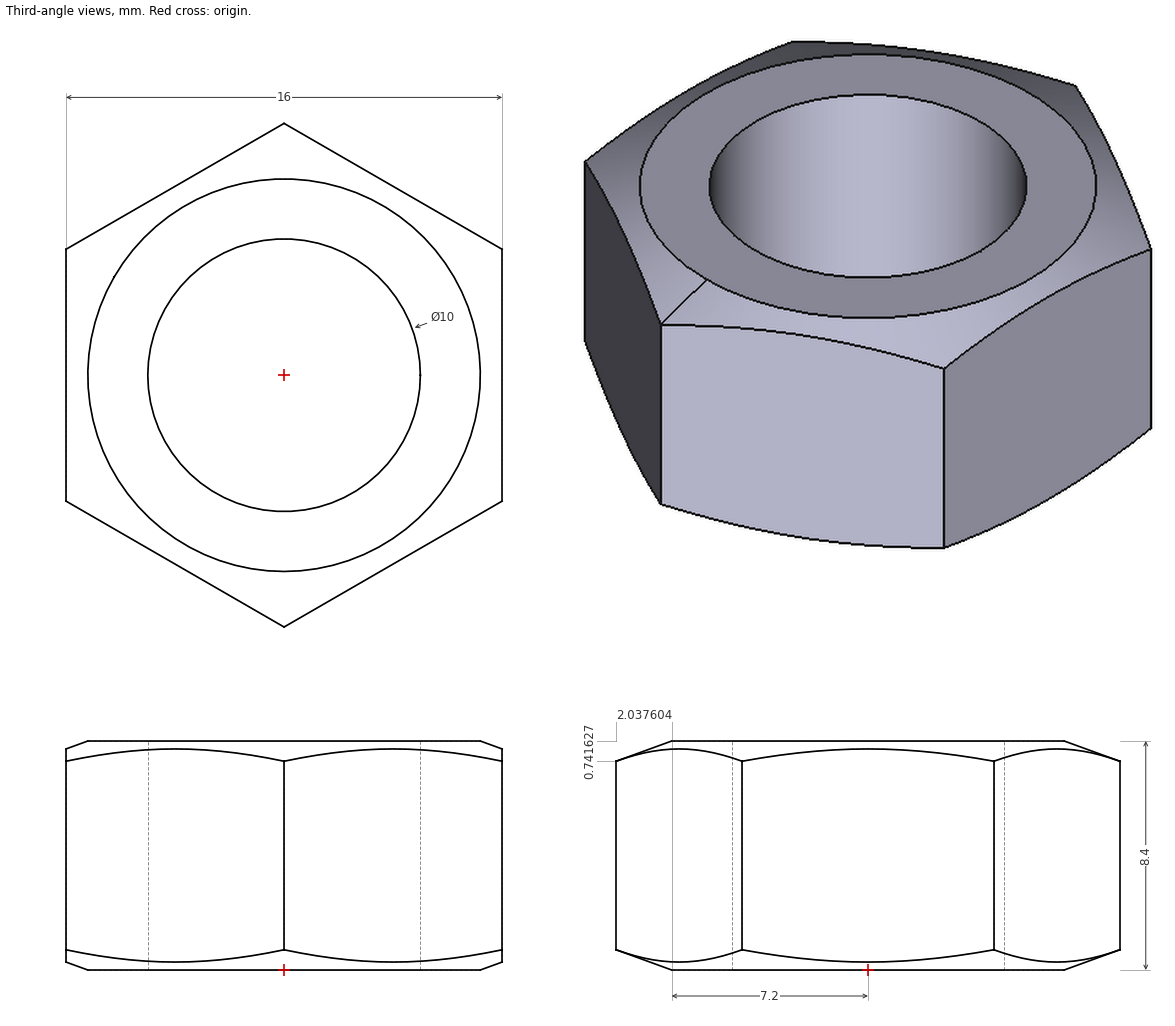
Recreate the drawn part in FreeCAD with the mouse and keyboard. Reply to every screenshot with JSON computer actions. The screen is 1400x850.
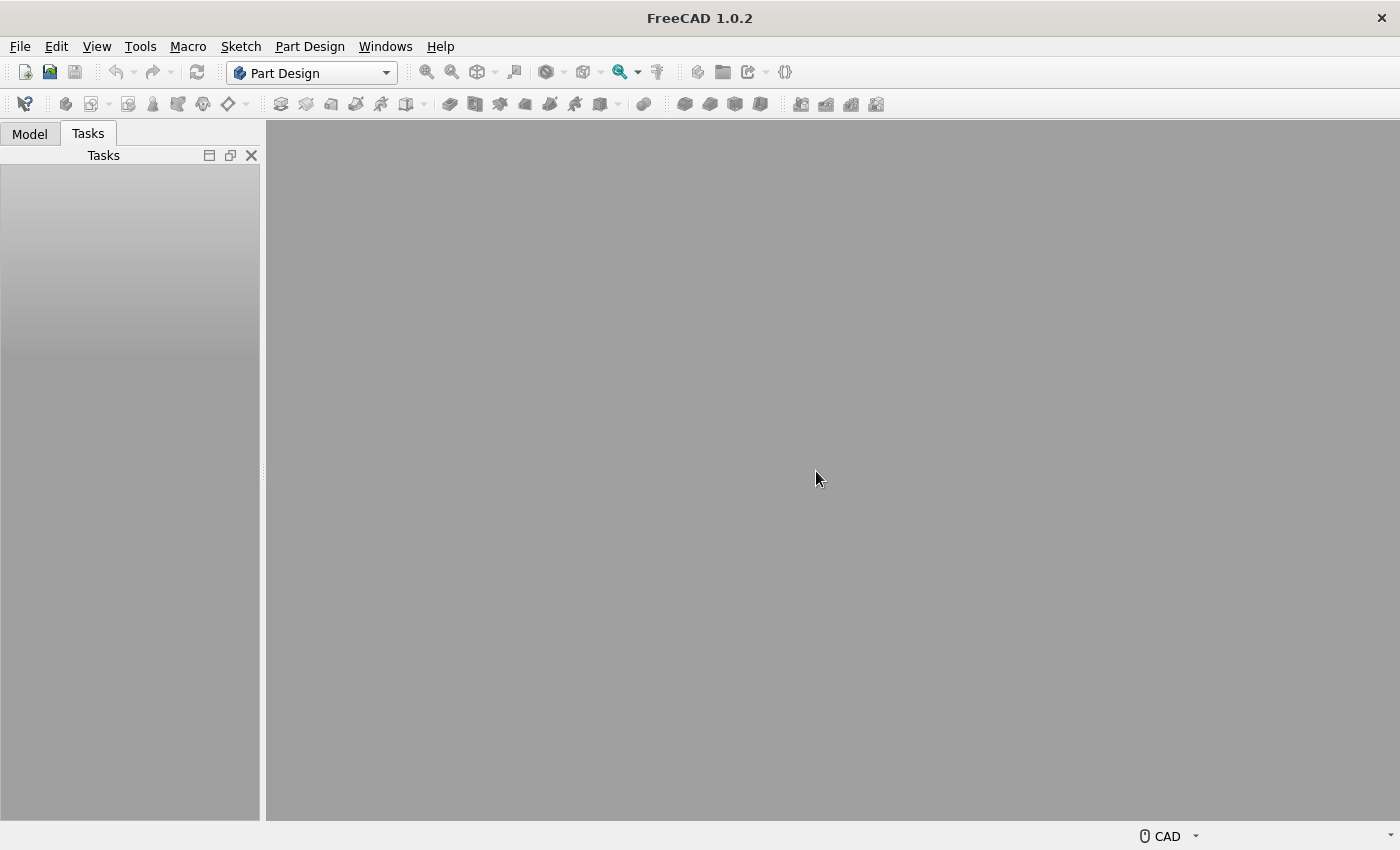
{"action": "left_click", "coordinate": [25, 72]}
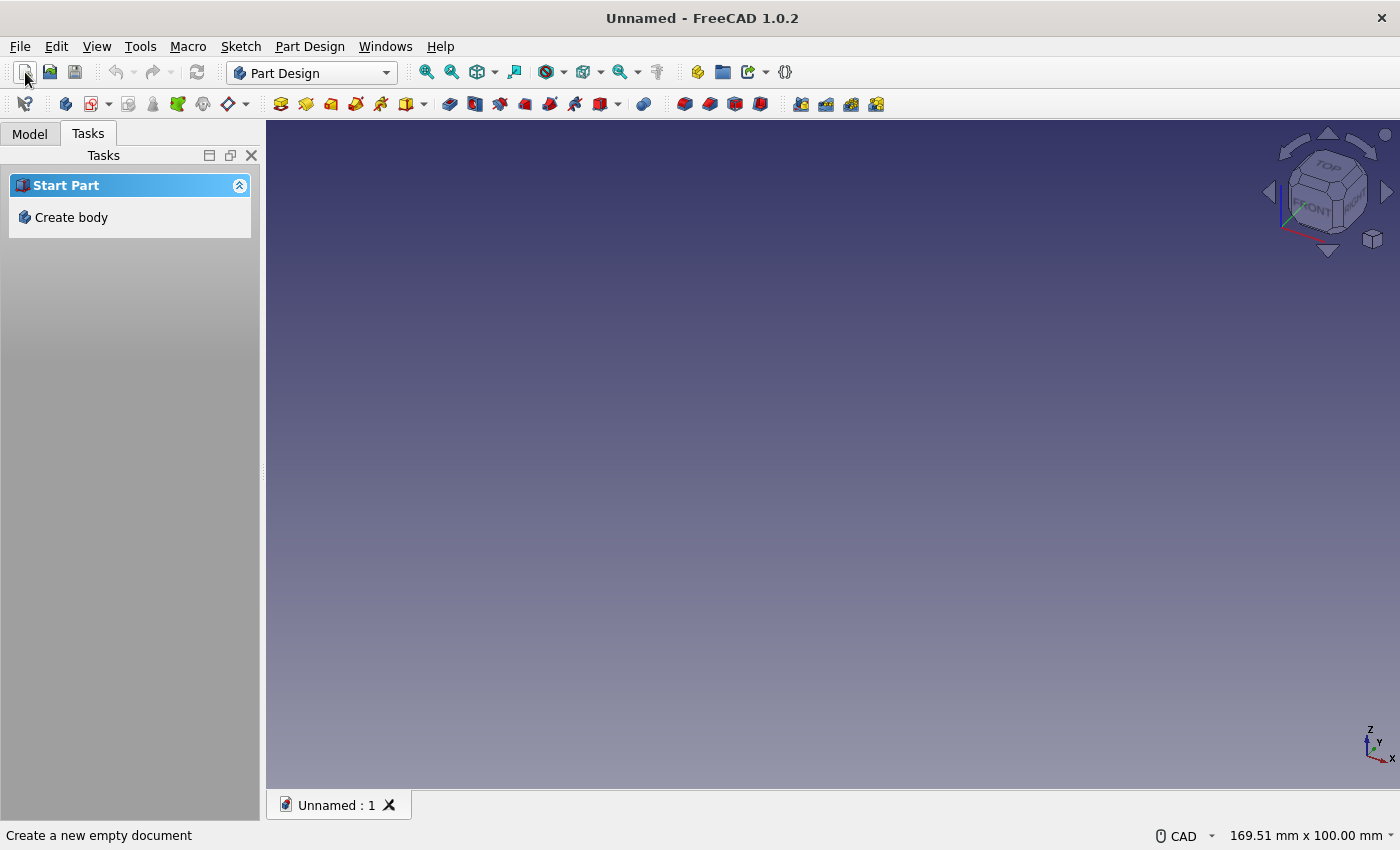
{"action": "left_click", "coordinate": [90, 104]}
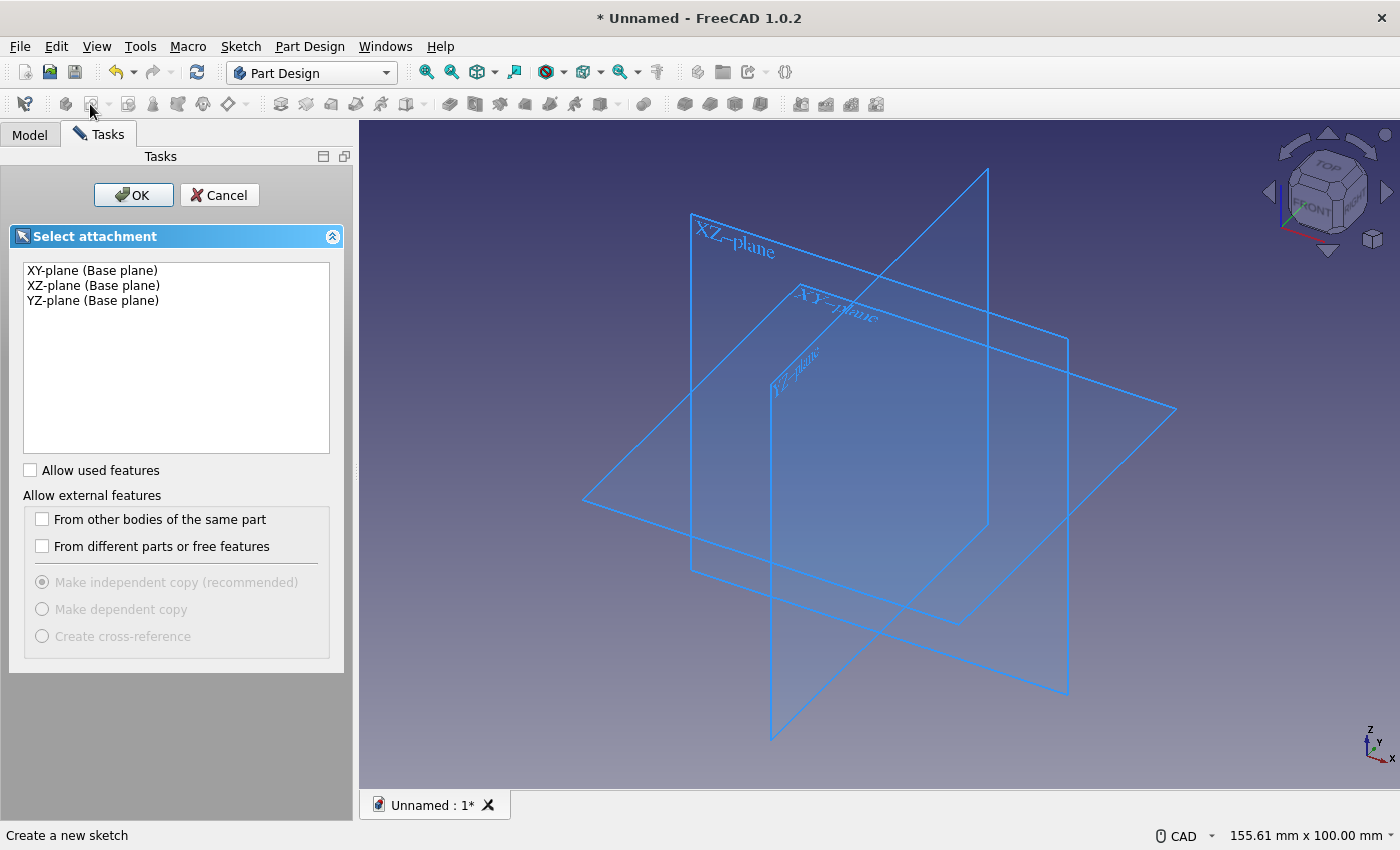
{"action": "left_click", "coordinate": [84, 270]}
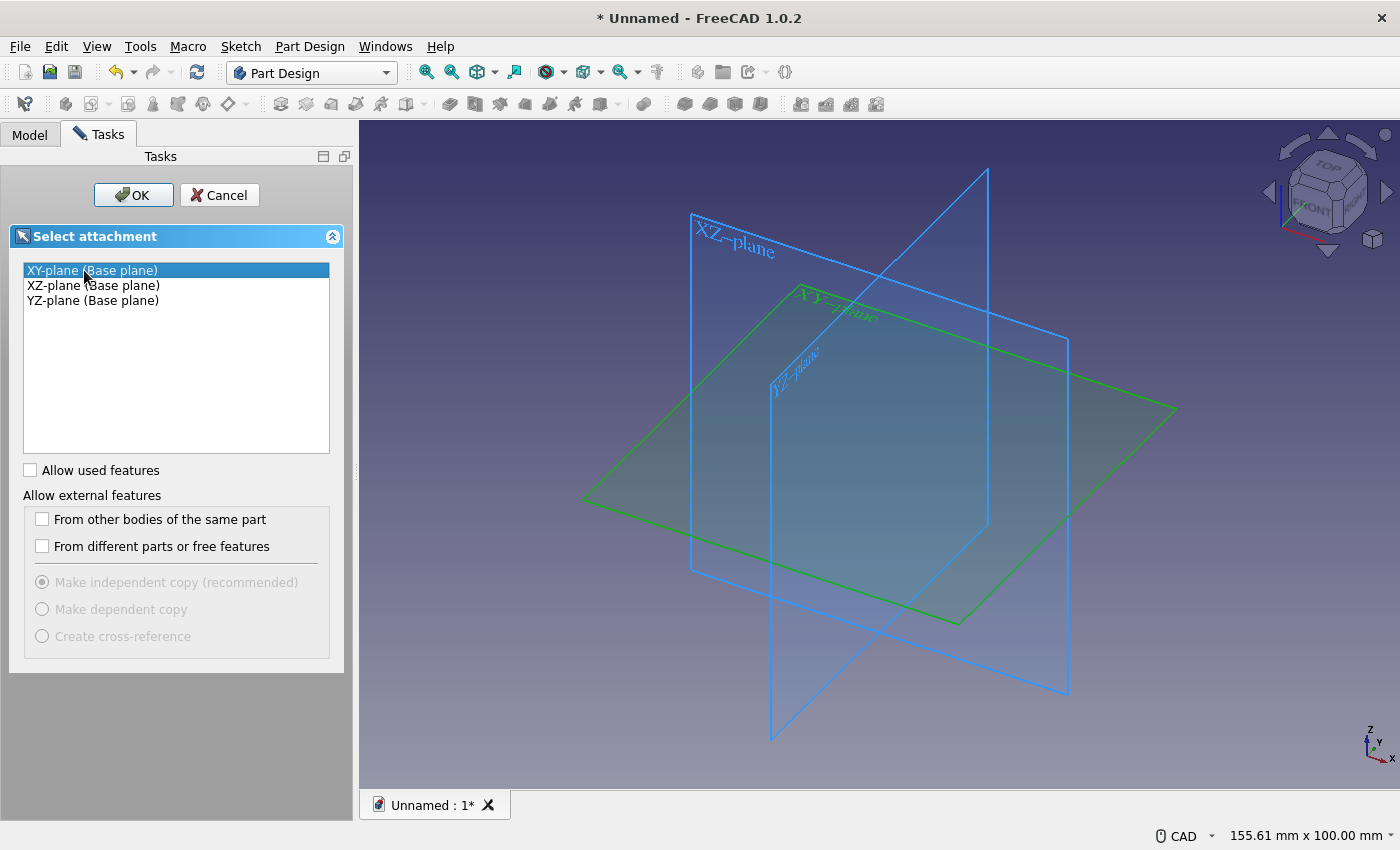
{"action": "left_click", "coordinate": [134, 195]}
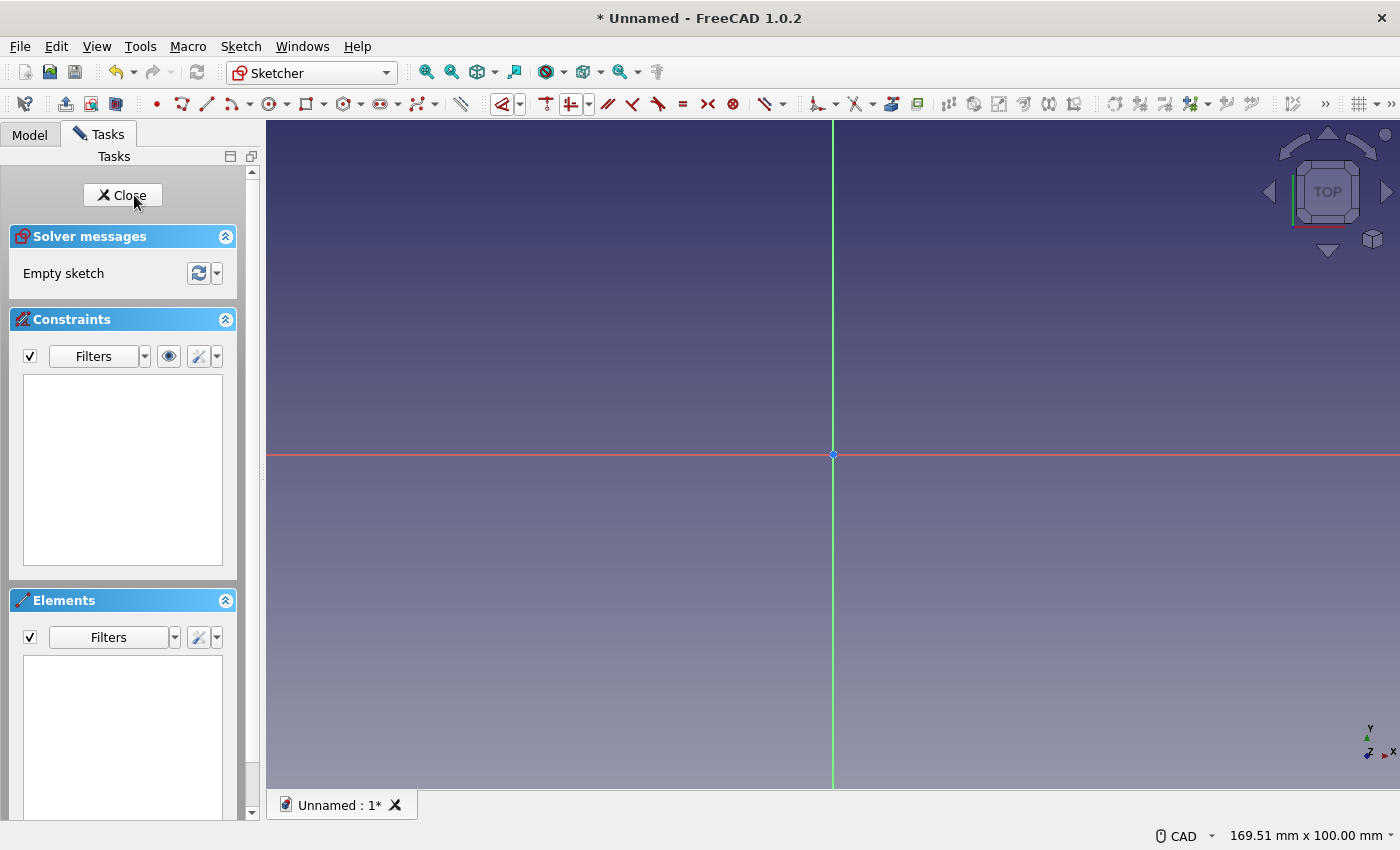
{"action": "scroll", "coordinate": [863, 455], "scroll_direction": "up", "scroll_amount": 6}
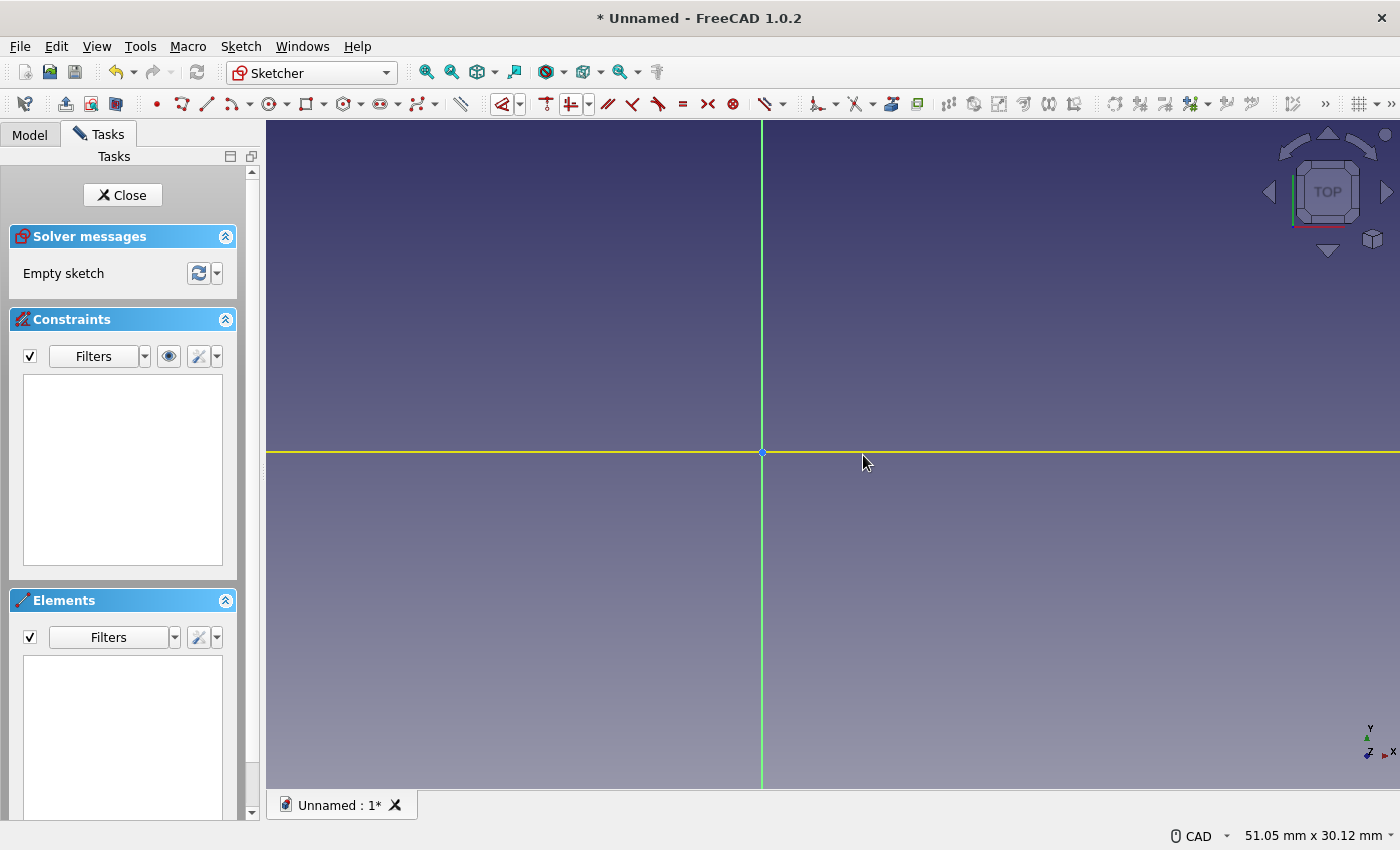
{"action": "key", "text": "g p 6"}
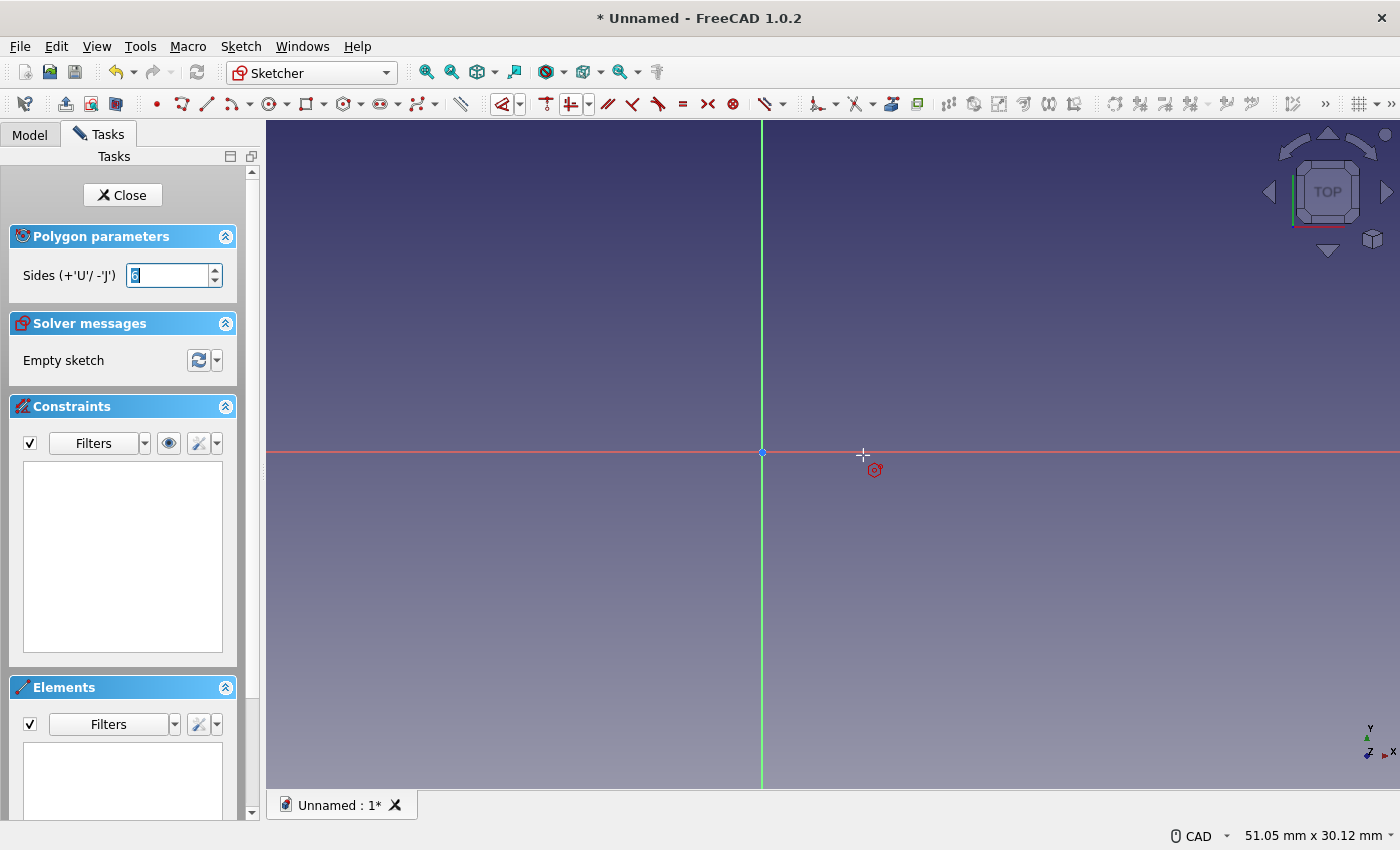
{"action": "left_click", "coordinate": [762, 452]}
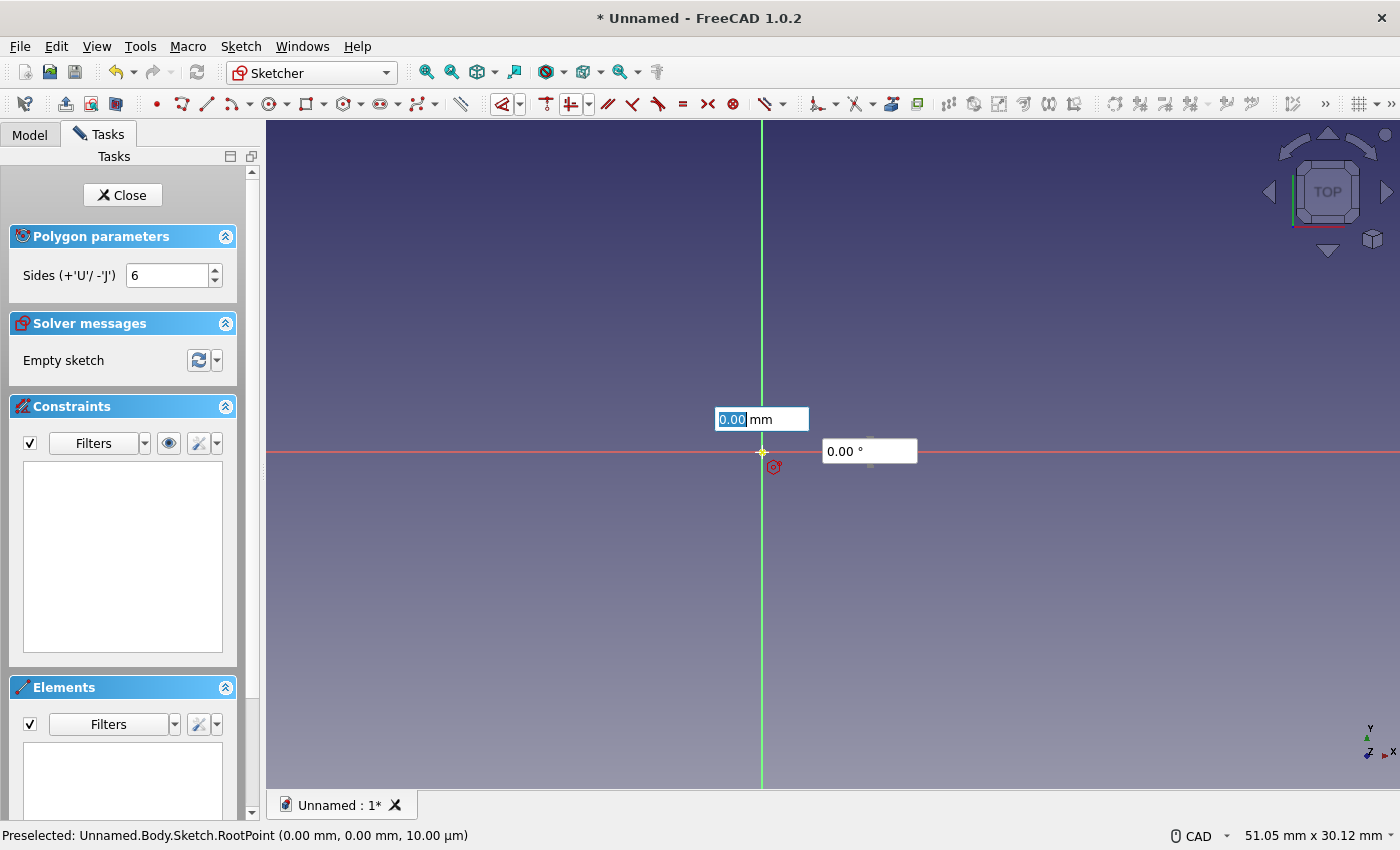
{"action": "left_click", "coordinate": [762, 247]}
{"action": "right_click", "coordinate": [762, 247]}